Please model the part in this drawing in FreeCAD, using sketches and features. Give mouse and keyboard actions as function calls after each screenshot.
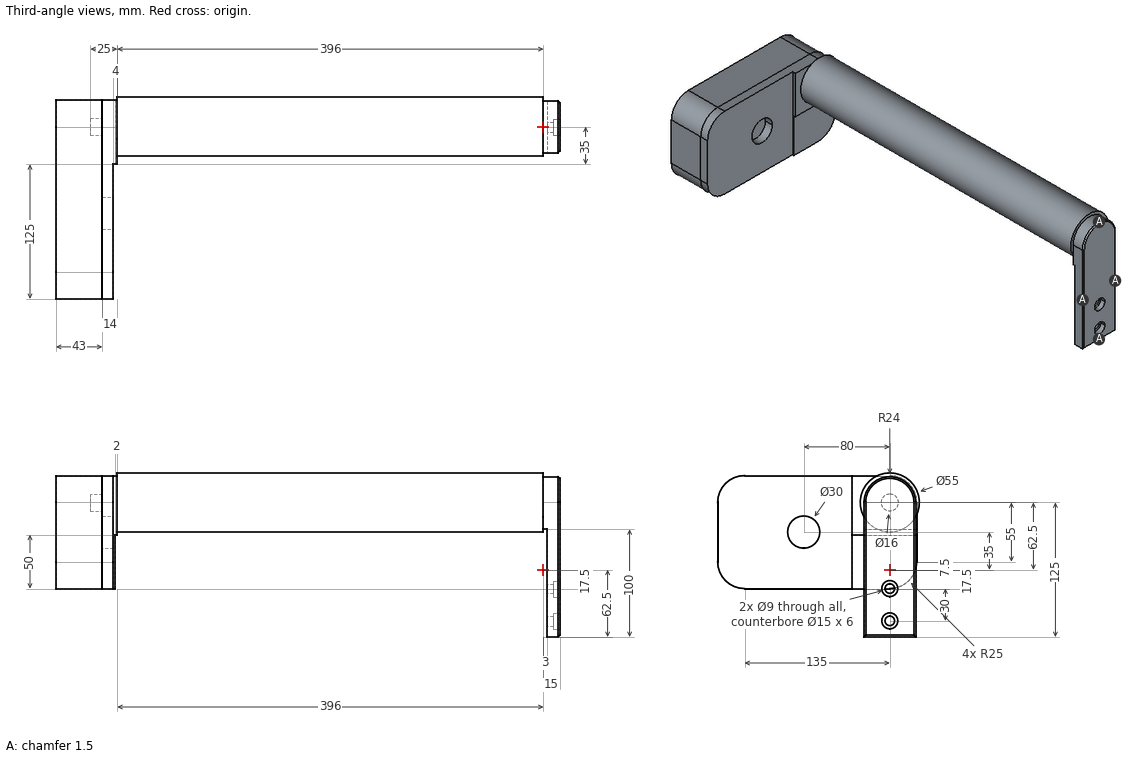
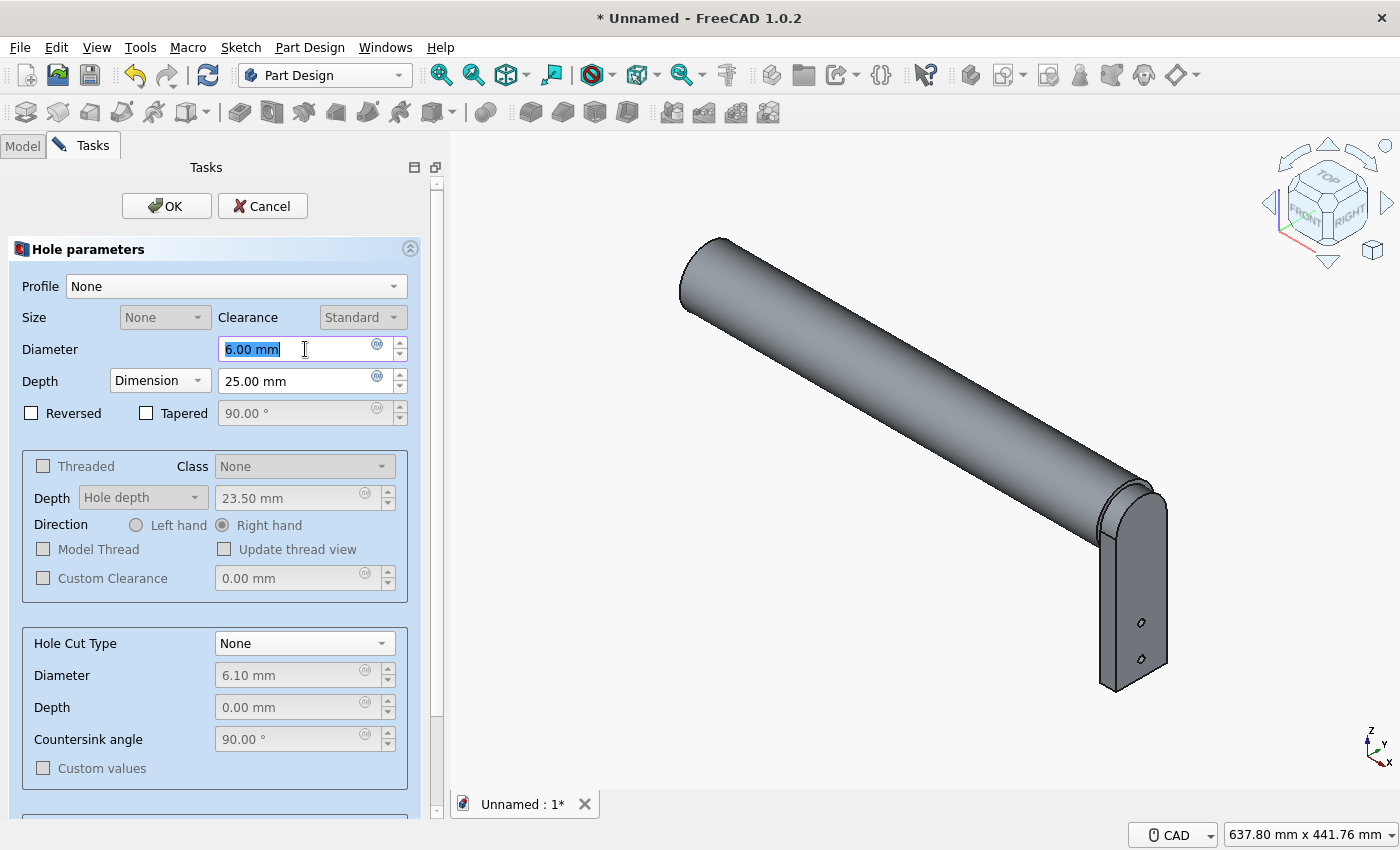
text(9)
key(Tab)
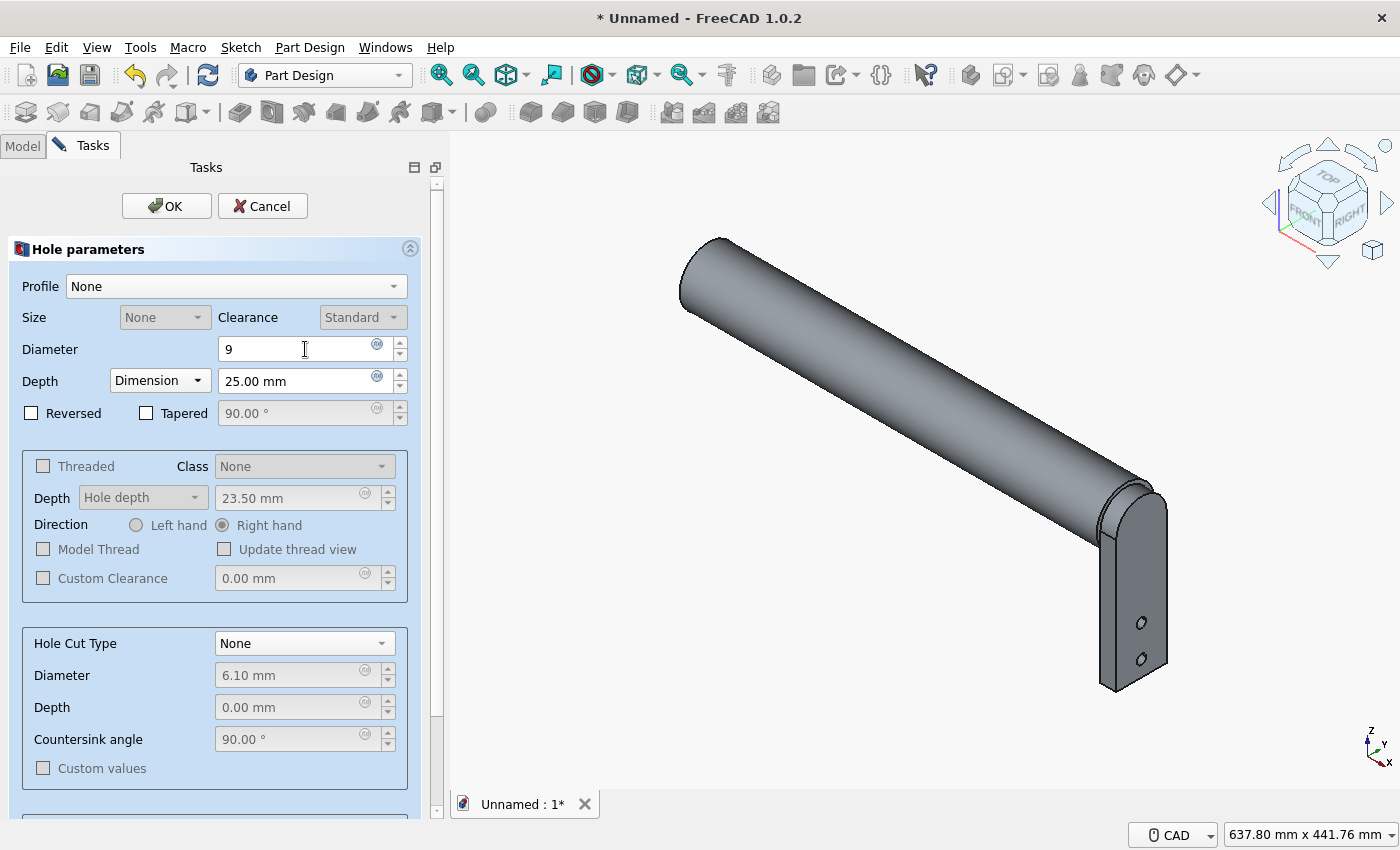
click(161, 380)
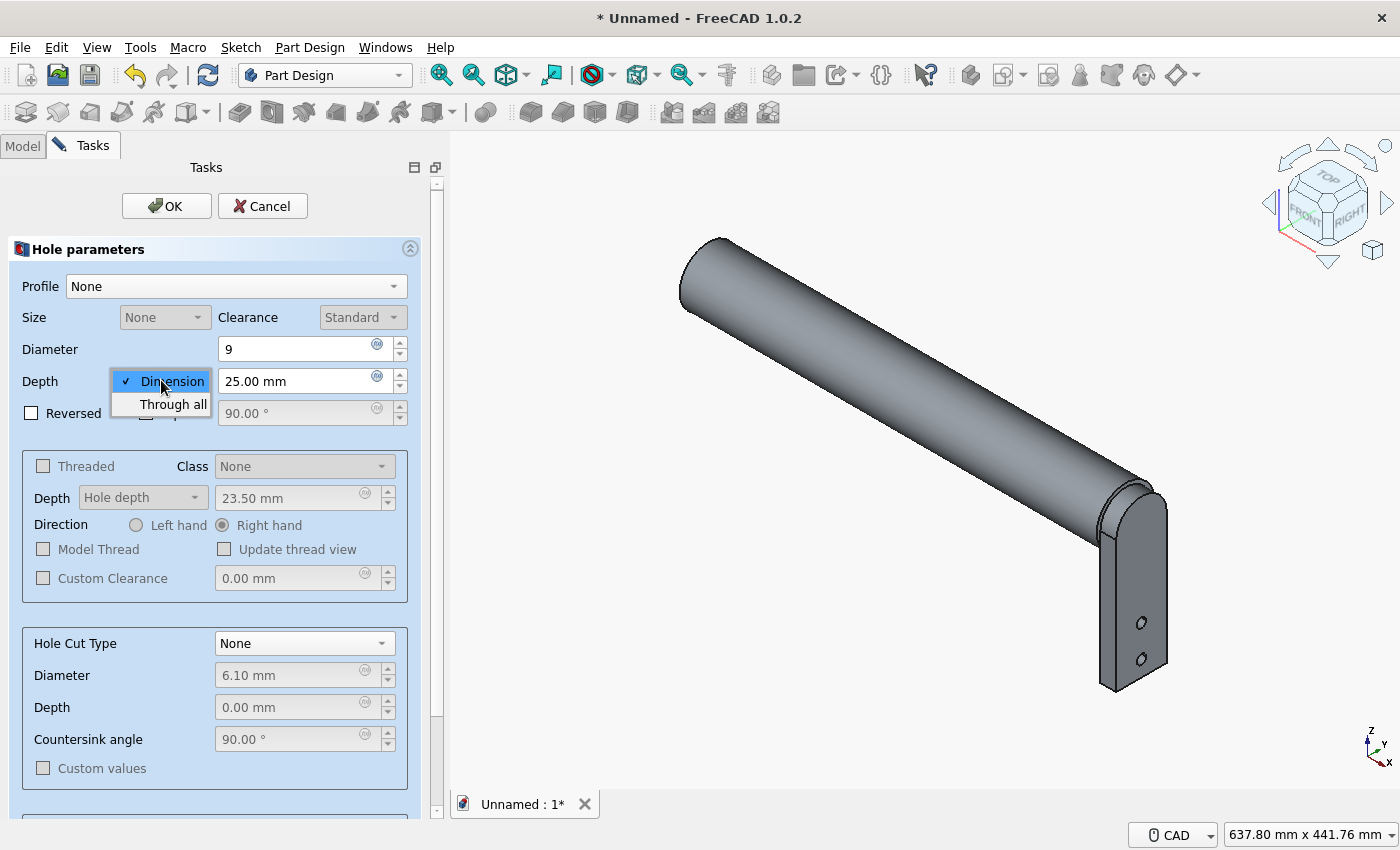
click(160, 404)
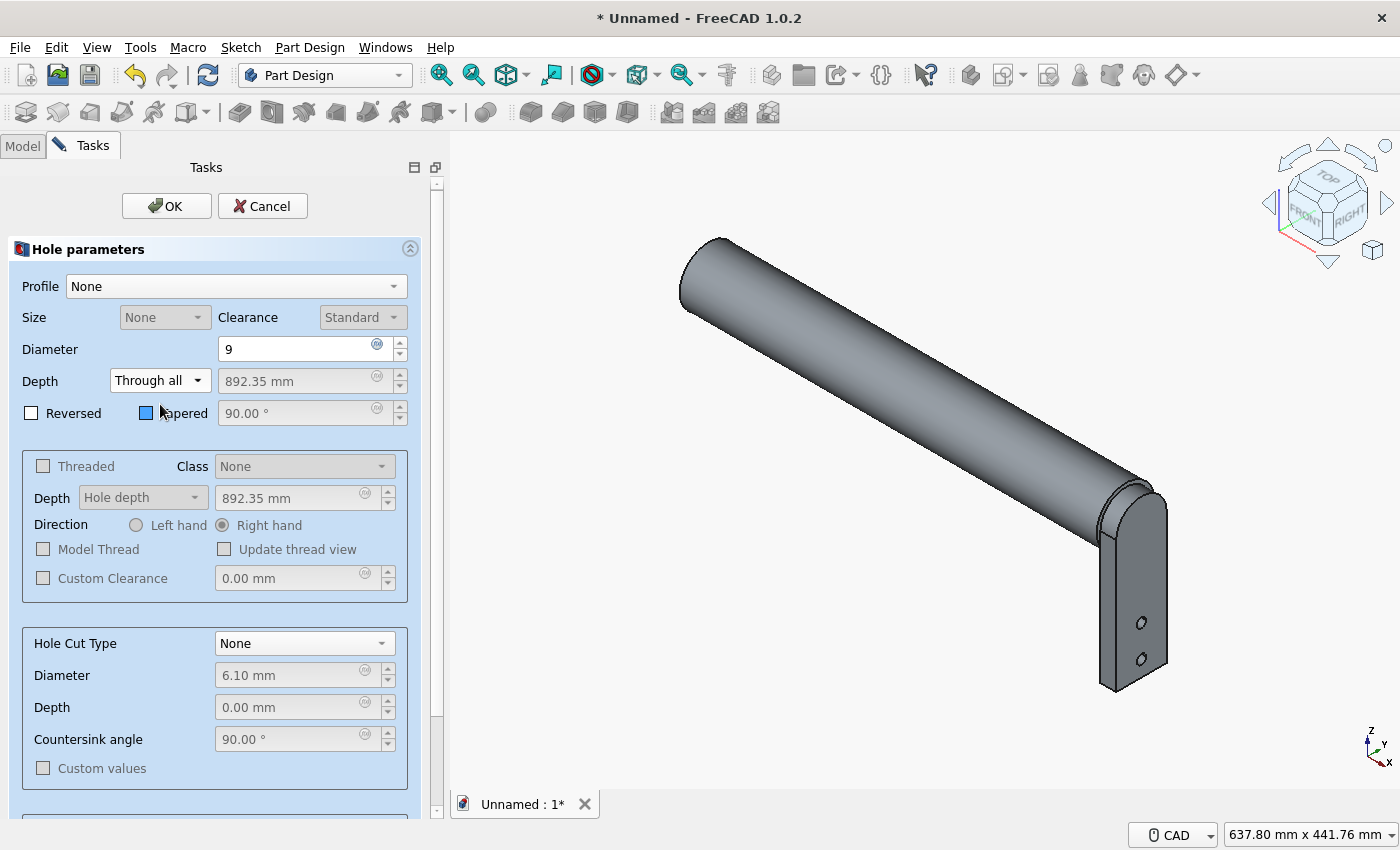
click(306, 644)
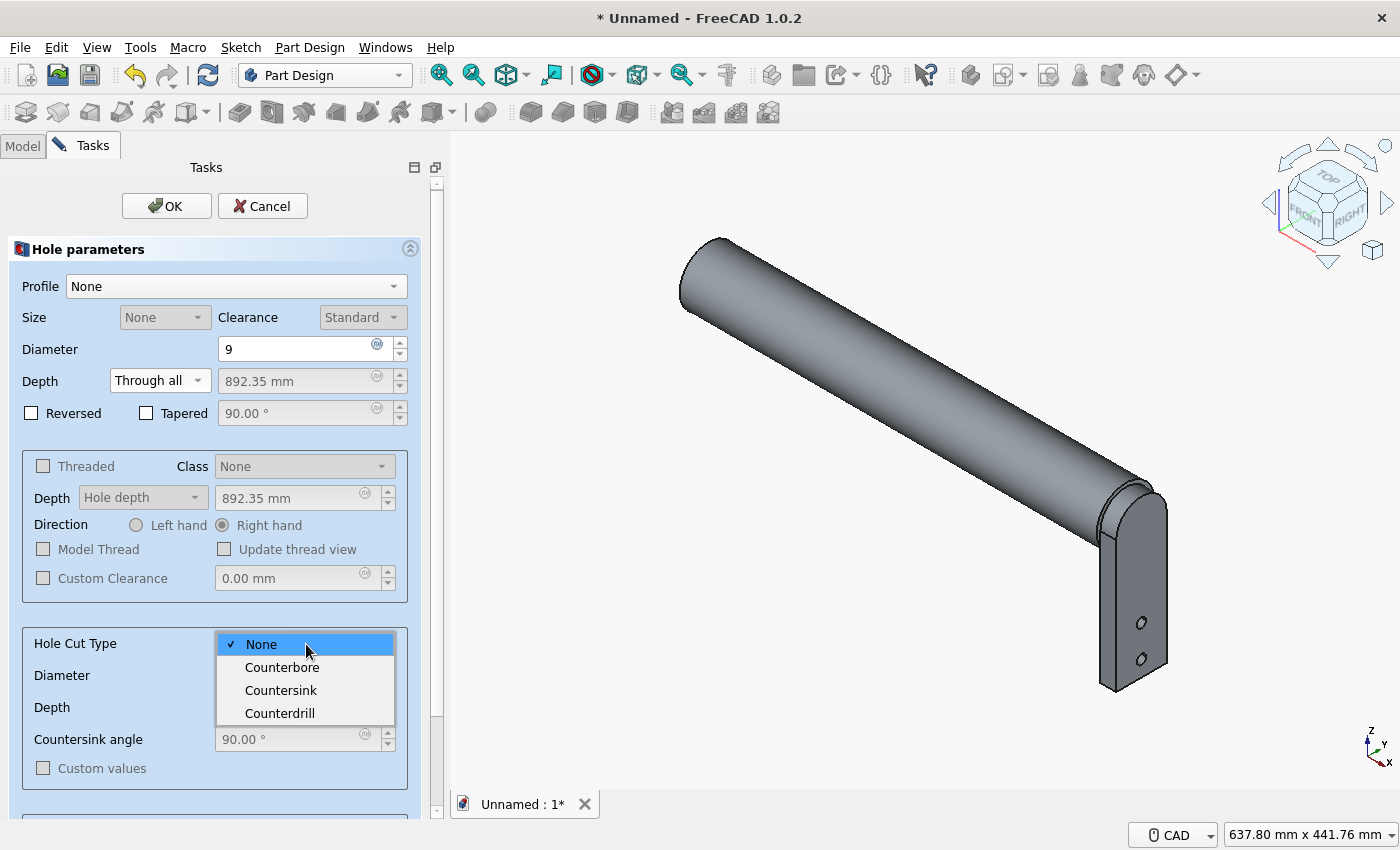
click(304, 668)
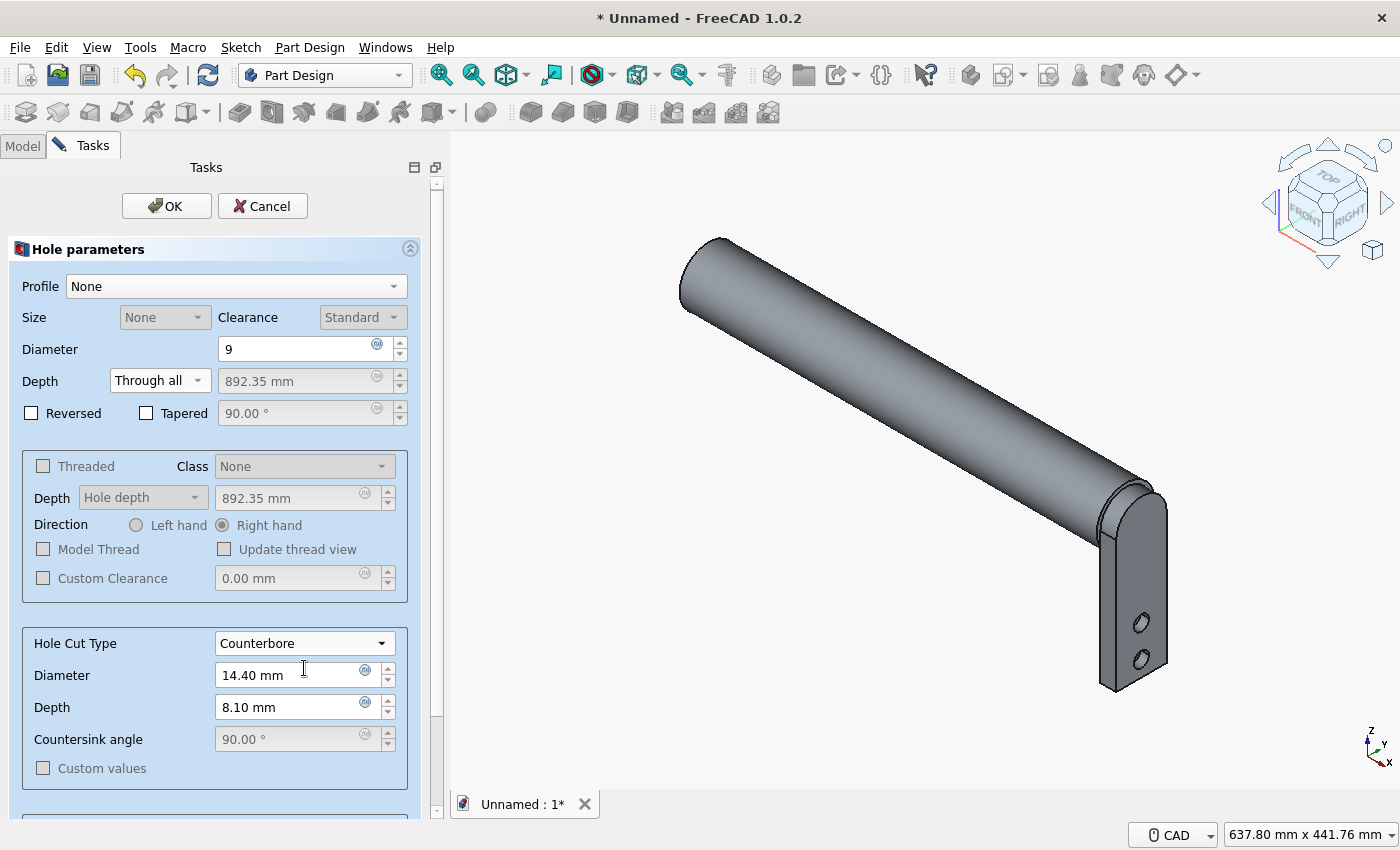
triple_click(298, 675)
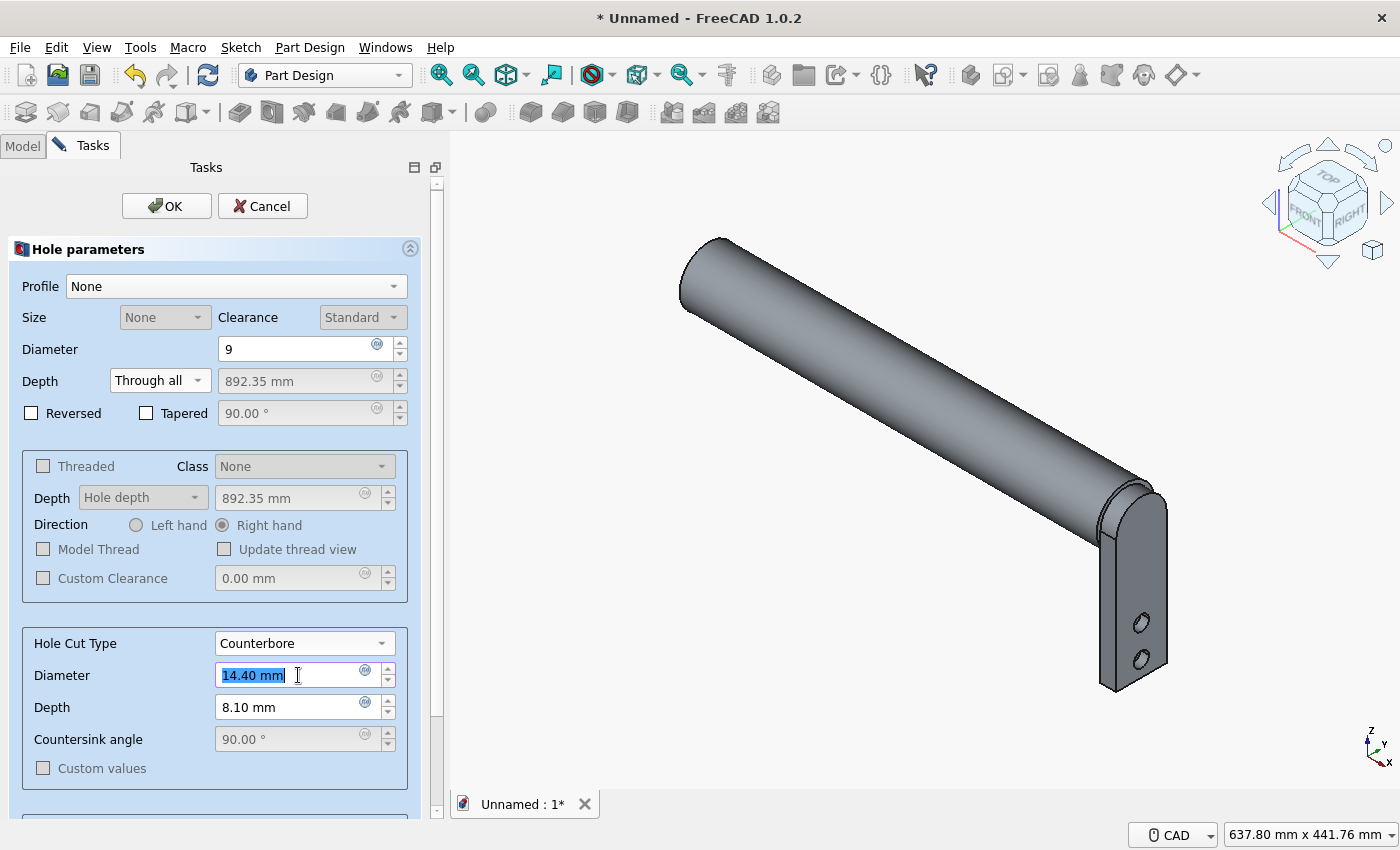
text(15)
key(Tab)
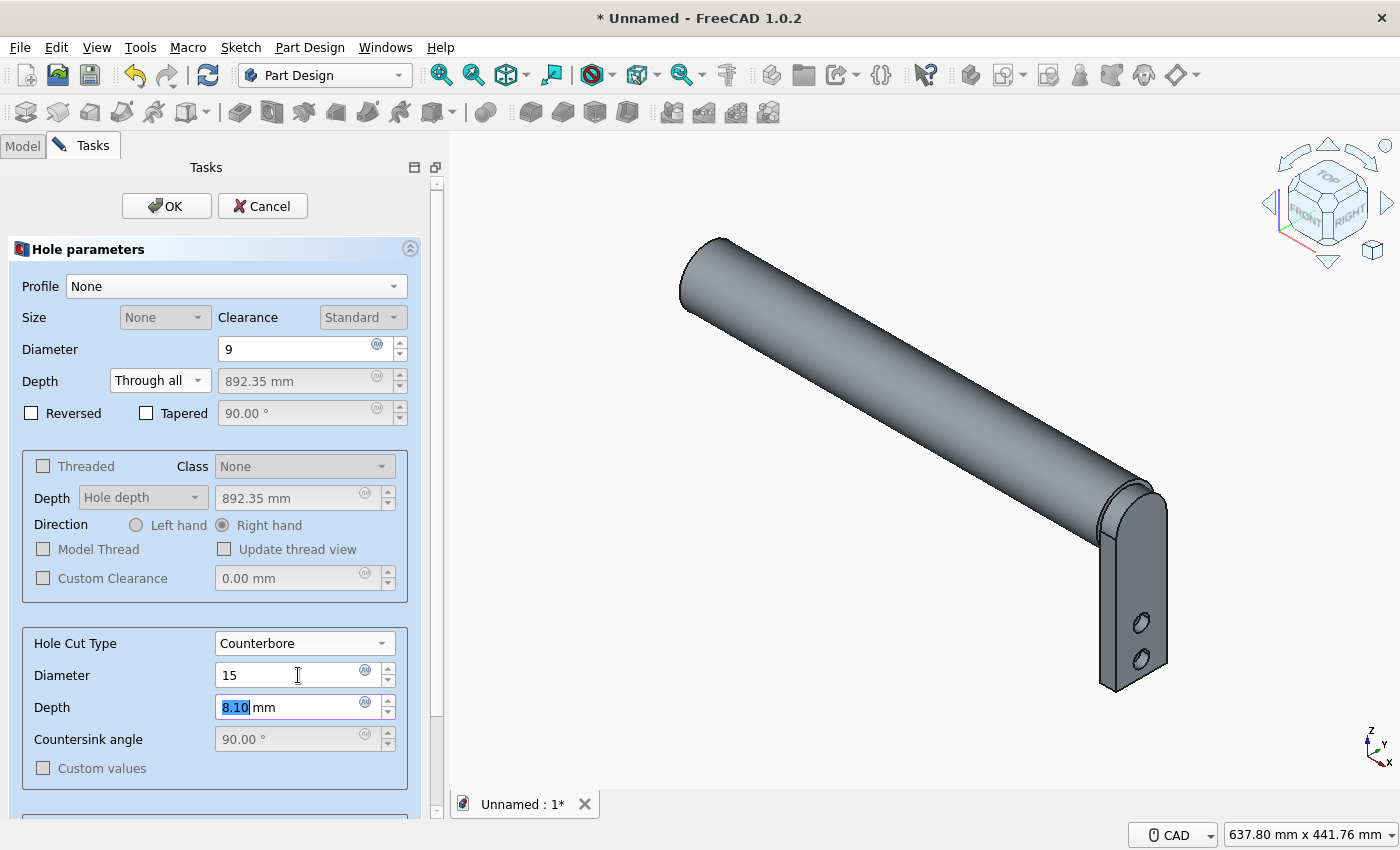
text(6)
key(Tab)